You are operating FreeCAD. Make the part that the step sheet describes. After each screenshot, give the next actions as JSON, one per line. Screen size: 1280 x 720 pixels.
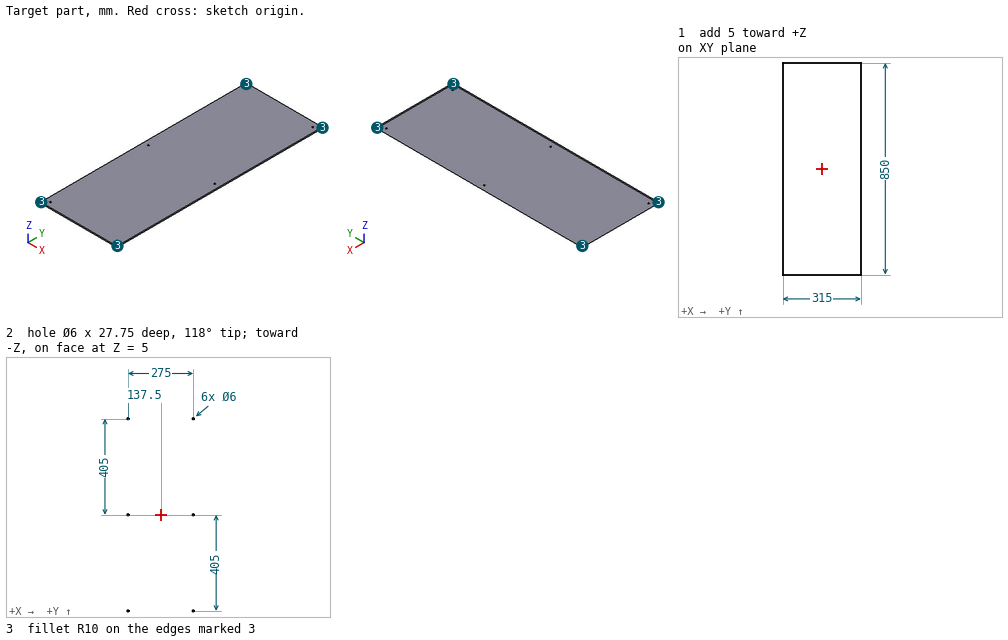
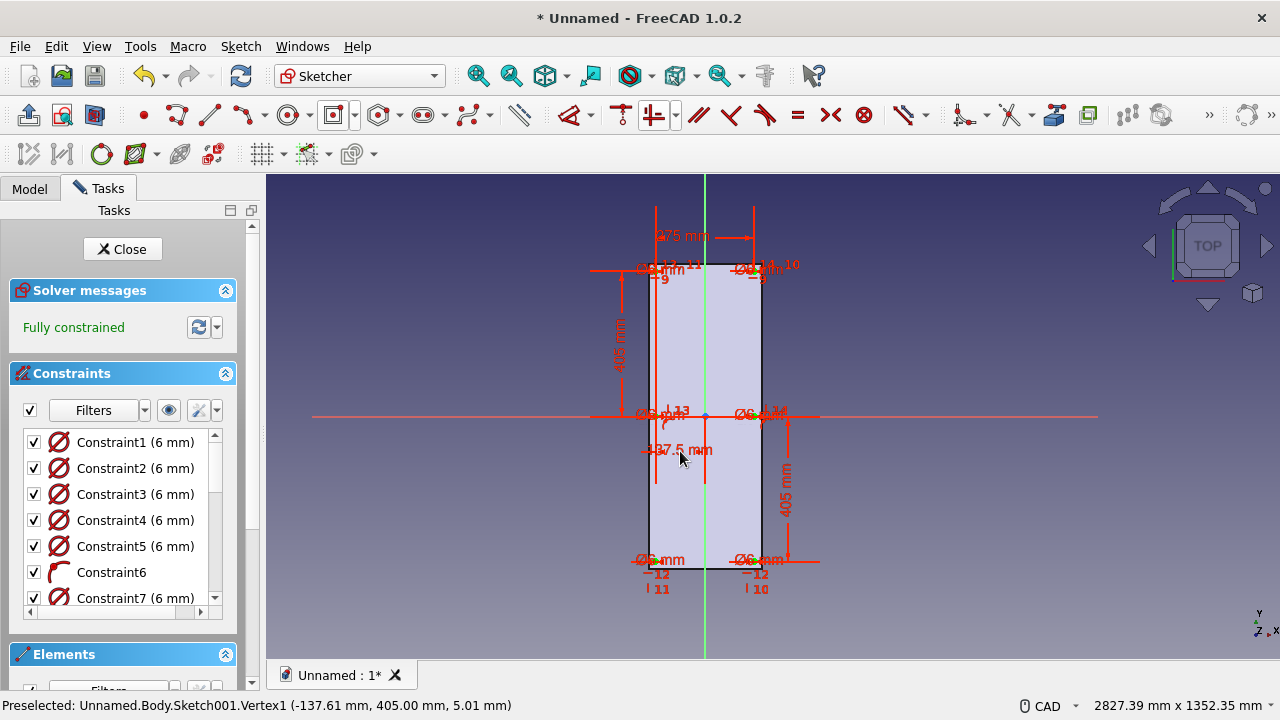
{"action": "left_click", "coordinate": [123, 249]}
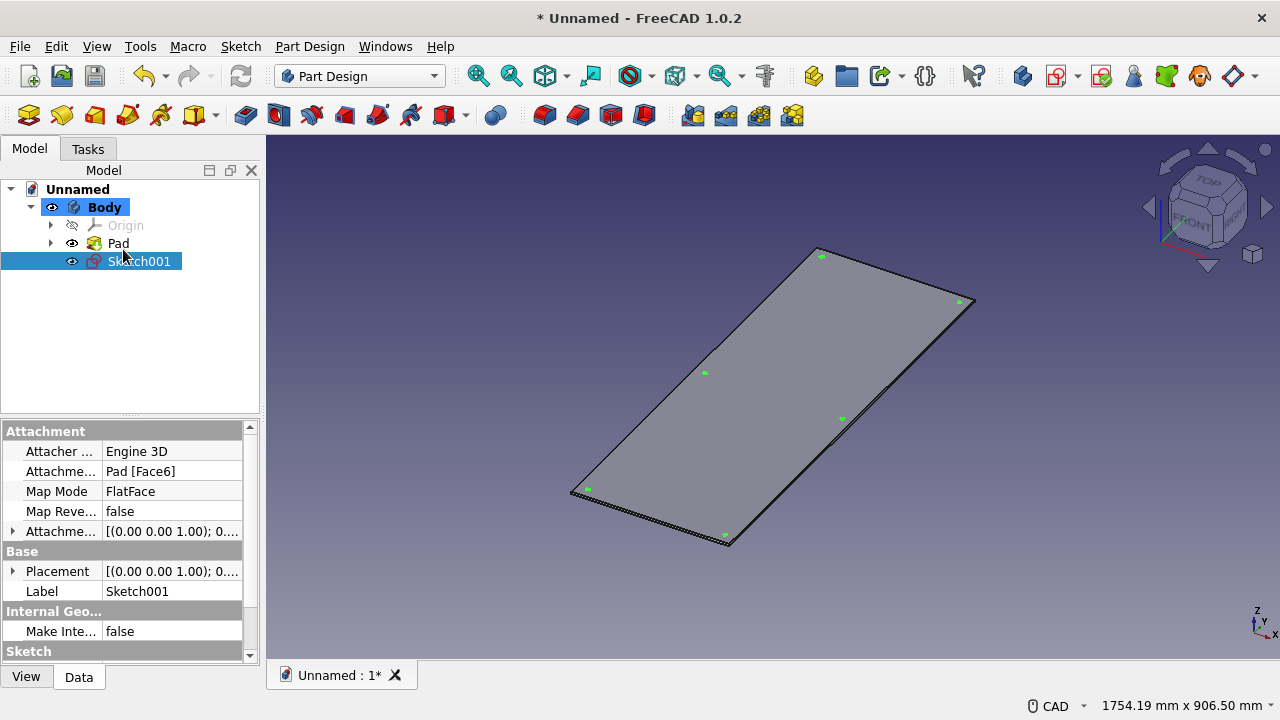
{"action": "left_click", "coordinate": [279, 116]}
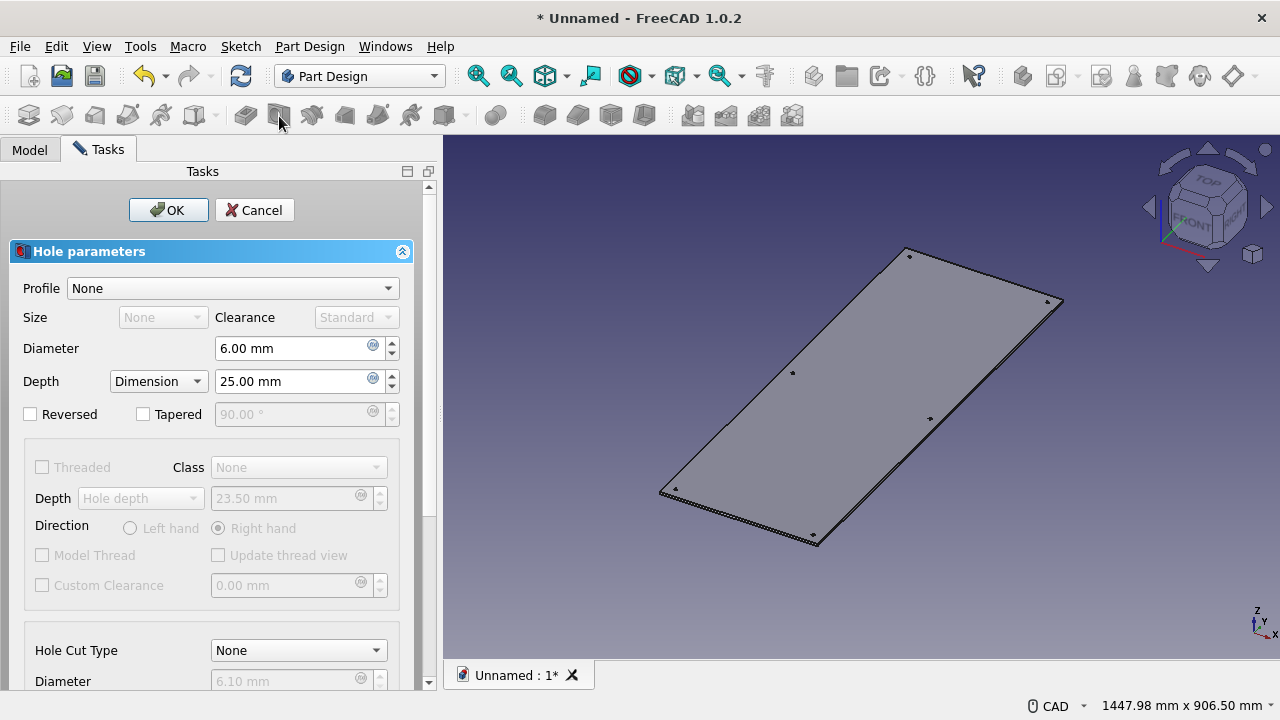
{"action": "triple_click", "coordinate": [300, 348]}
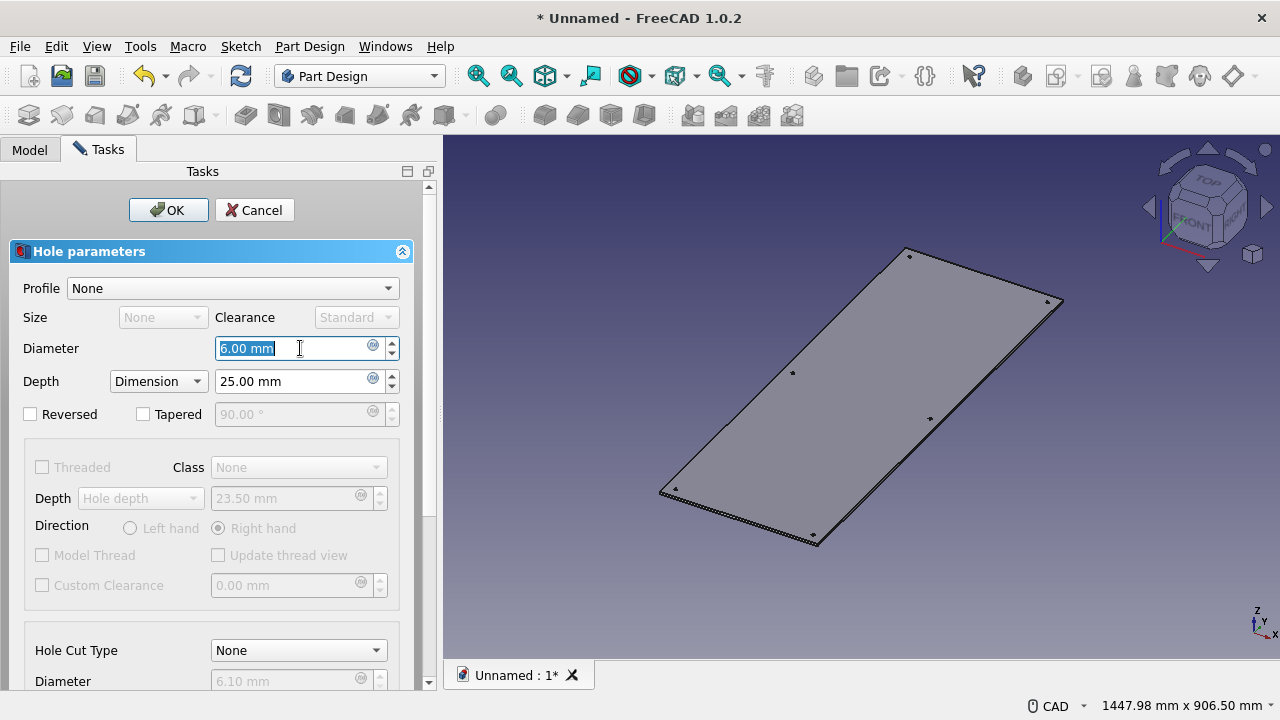
{"action": "type", "text": "6"}
{"action": "key", "text": "Tab"}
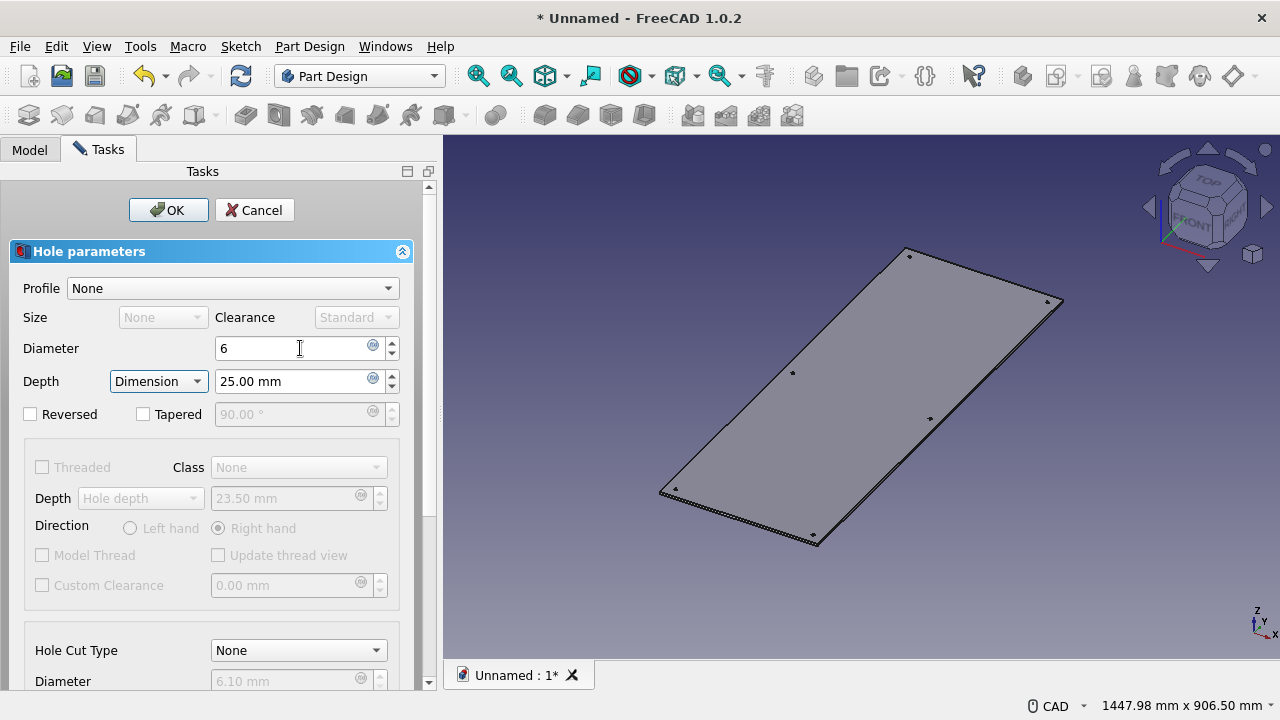
{"action": "triple_click", "coordinate": [300, 382]}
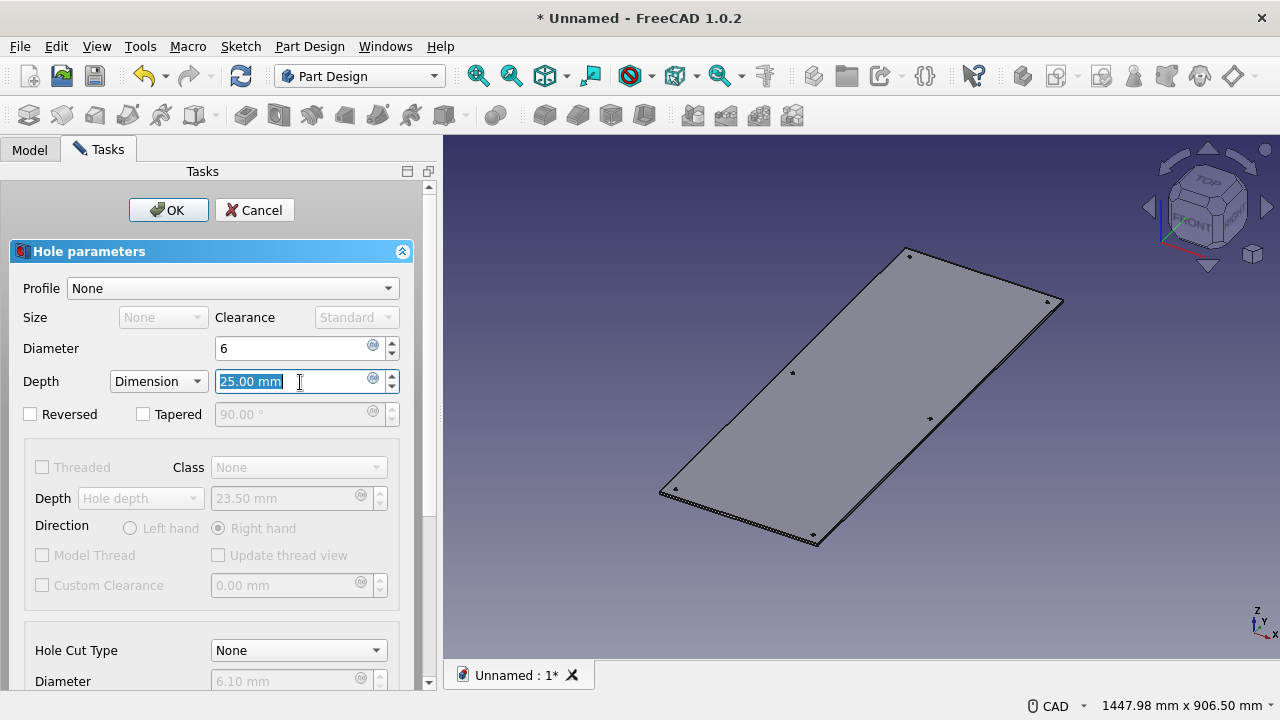
{"action": "type", "text": "27.75"}
{"action": "key", "text": "Tab"}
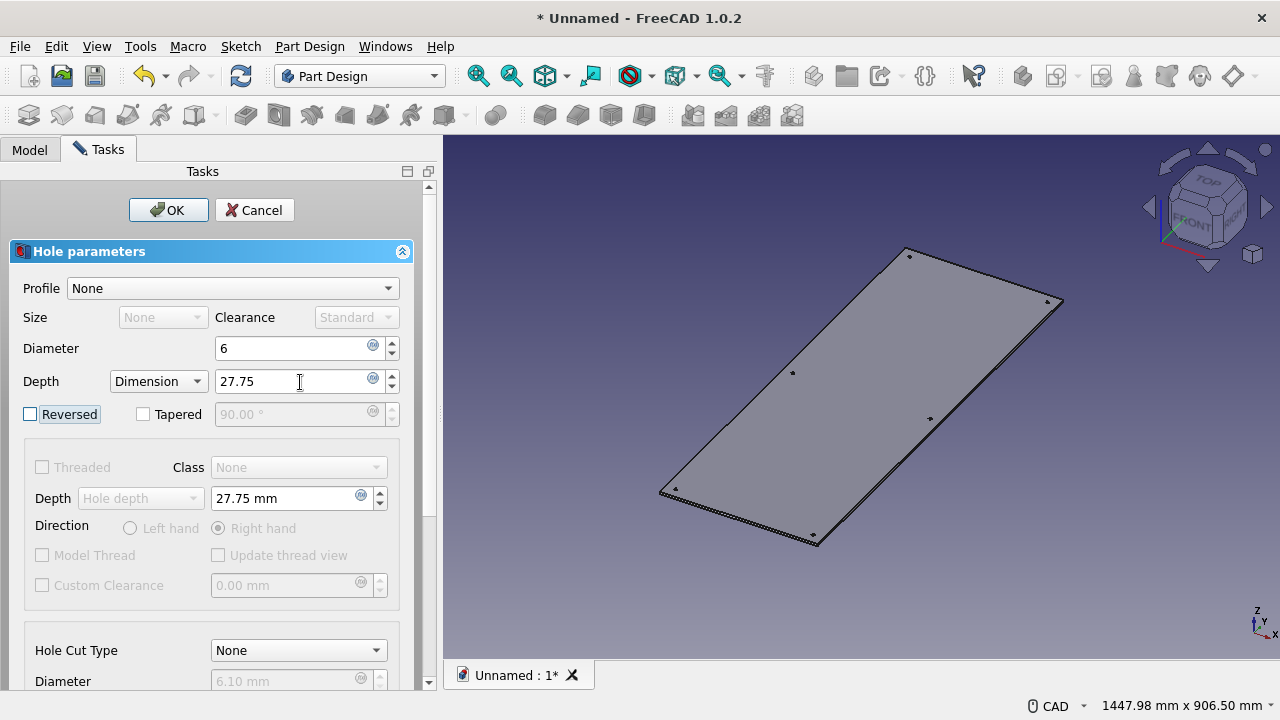
{"action": "left_click", "coordinate": [169, 210]}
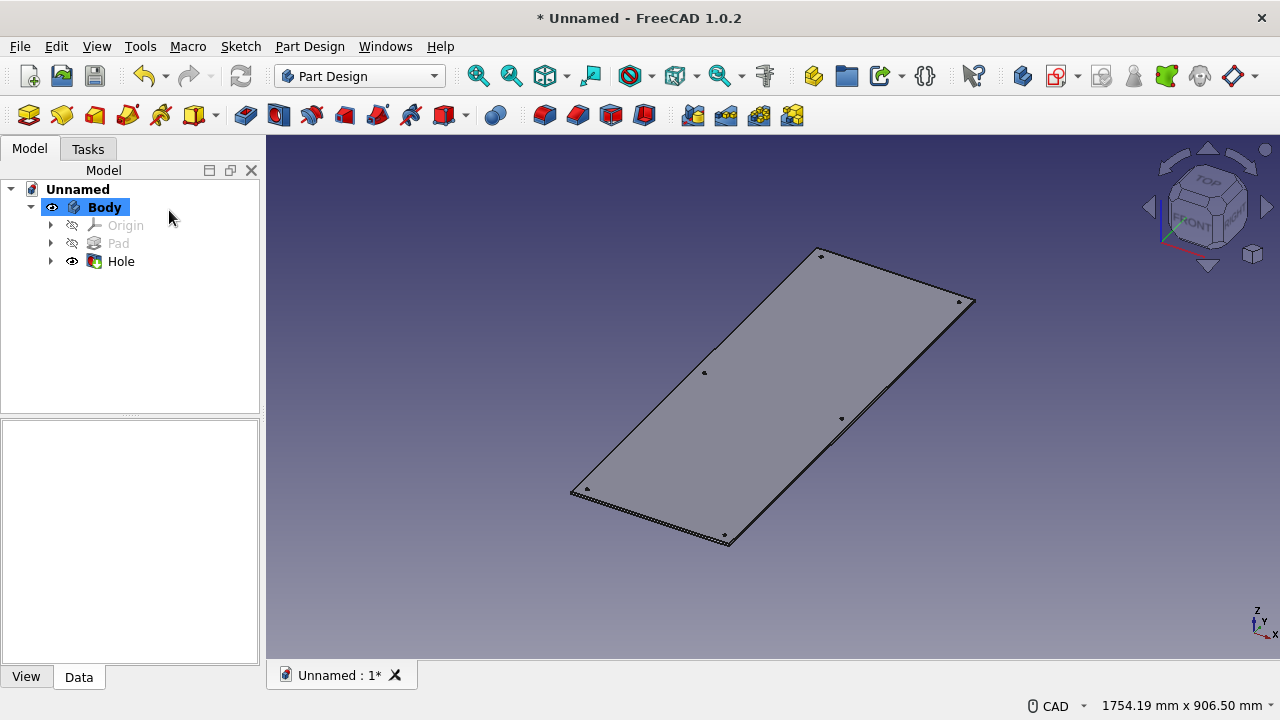
{"action": "scroll", "coordinate": [729, 544], "scroll_direction": "up", "scroll_amount": 14}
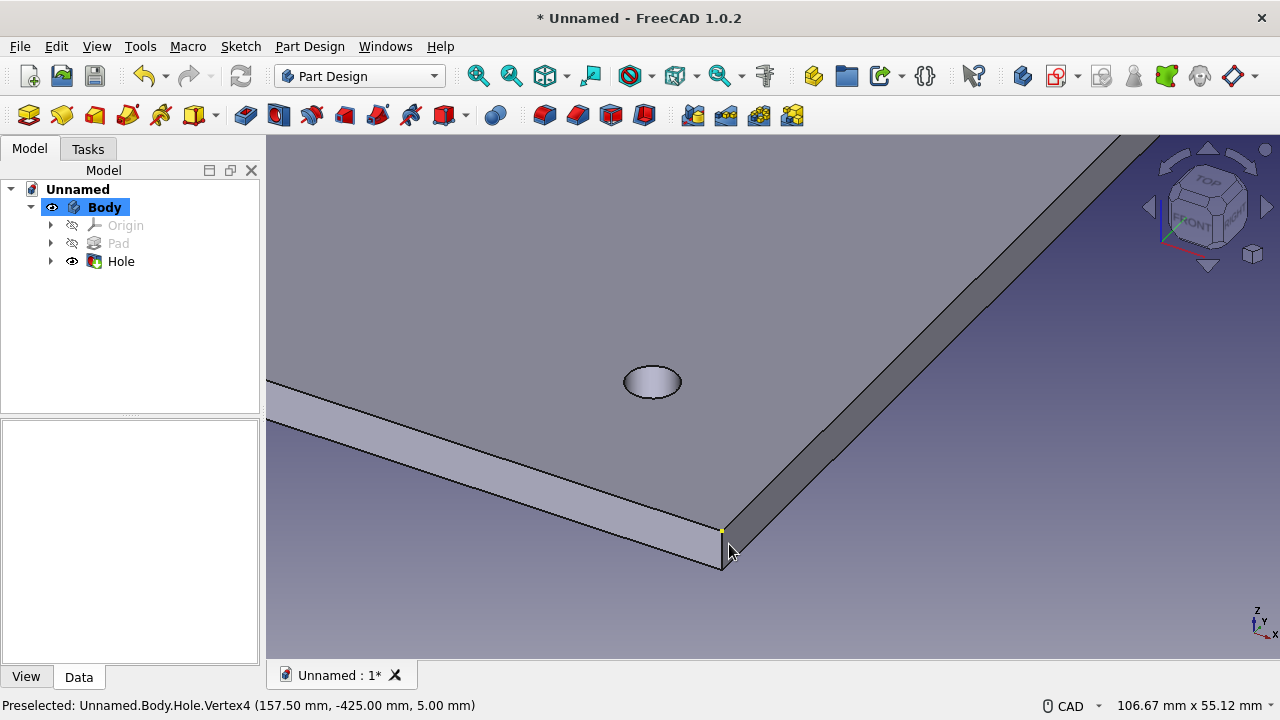
{"action": "left_click", "coordinate": [722, 550]}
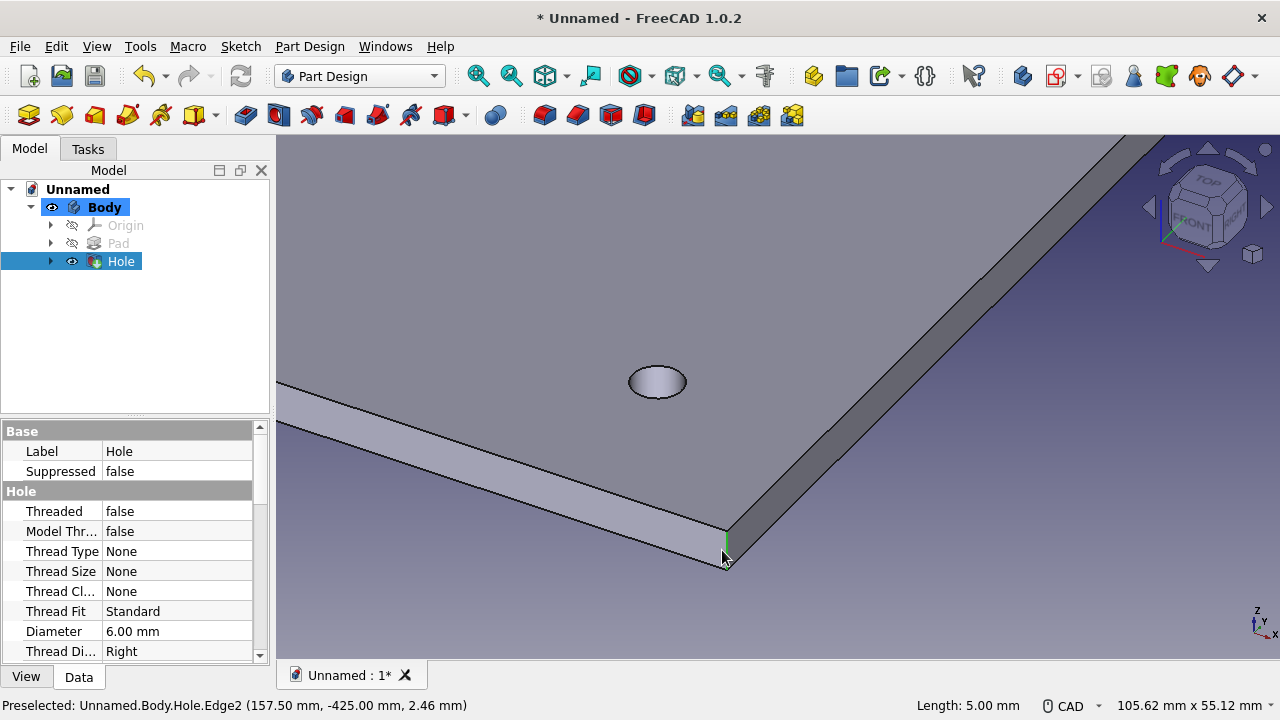
{"action": "left_click", "coordinate": [479, 76]}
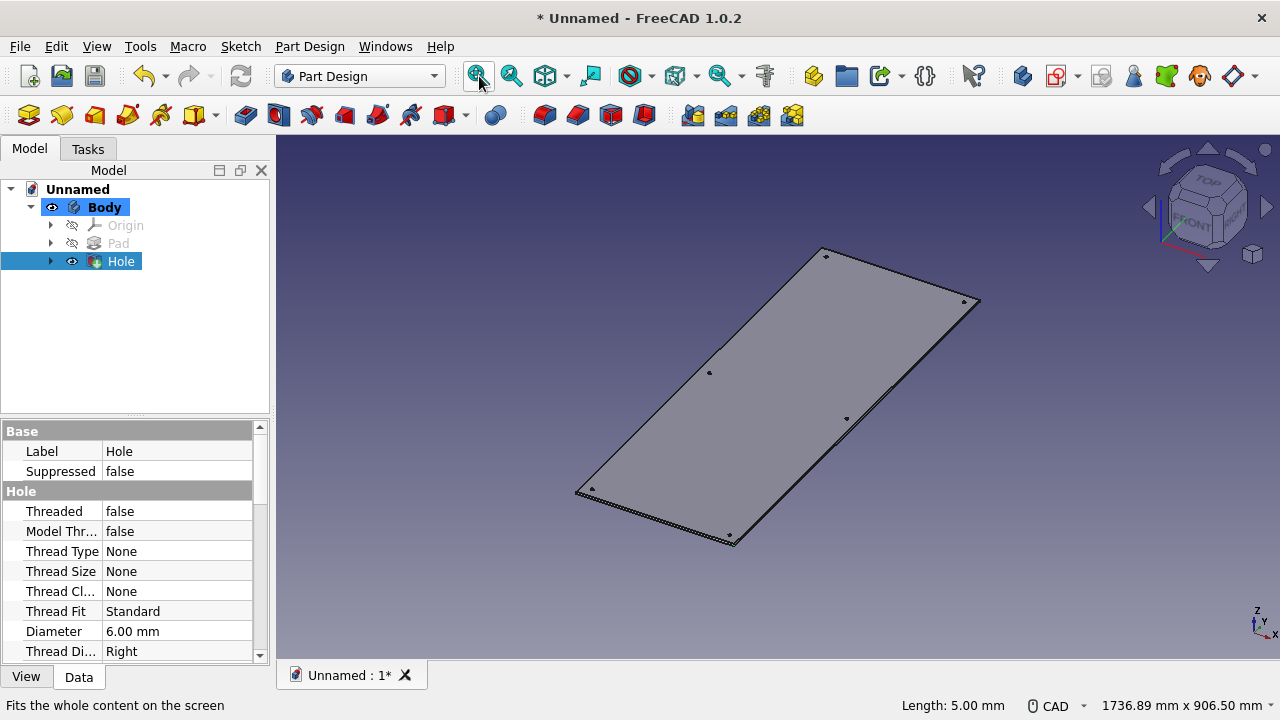
{"action": "key", "text": "0"}